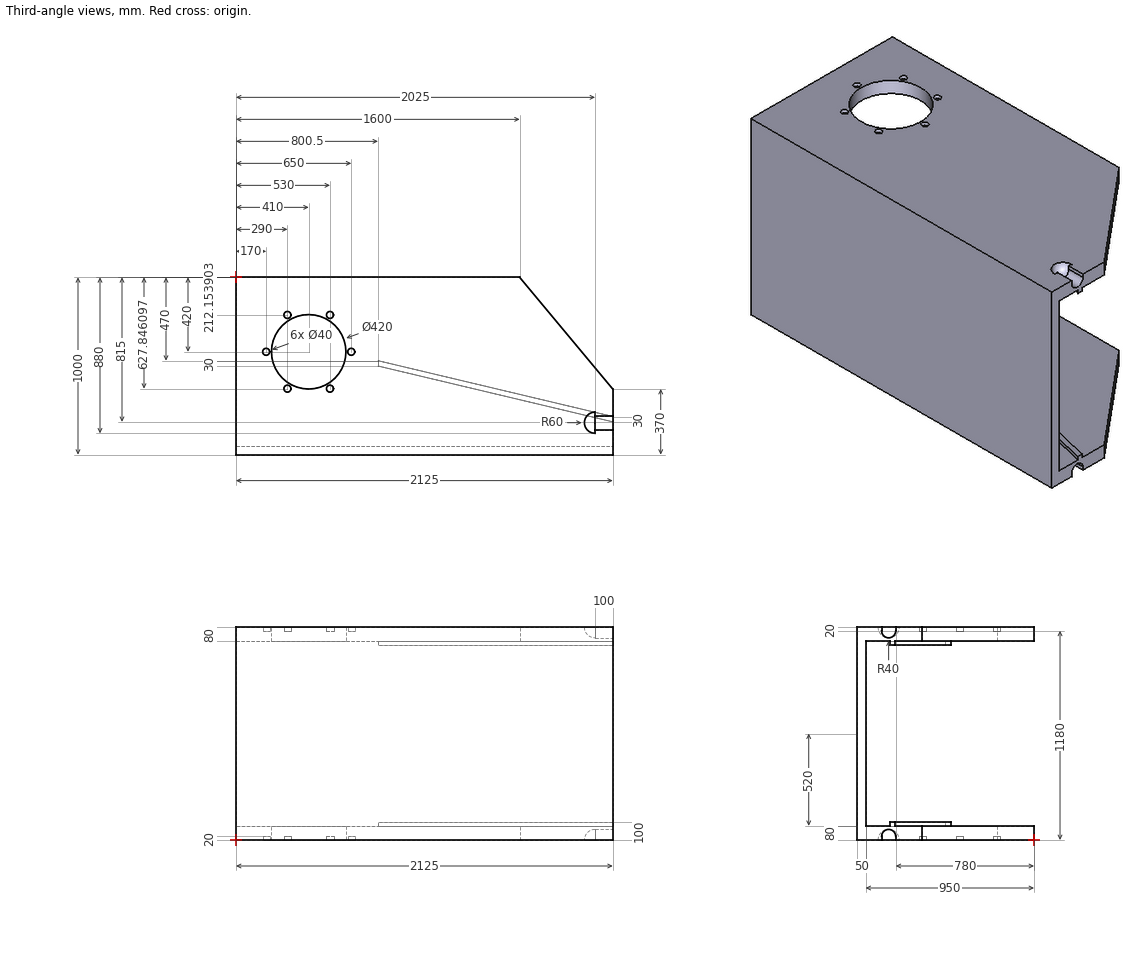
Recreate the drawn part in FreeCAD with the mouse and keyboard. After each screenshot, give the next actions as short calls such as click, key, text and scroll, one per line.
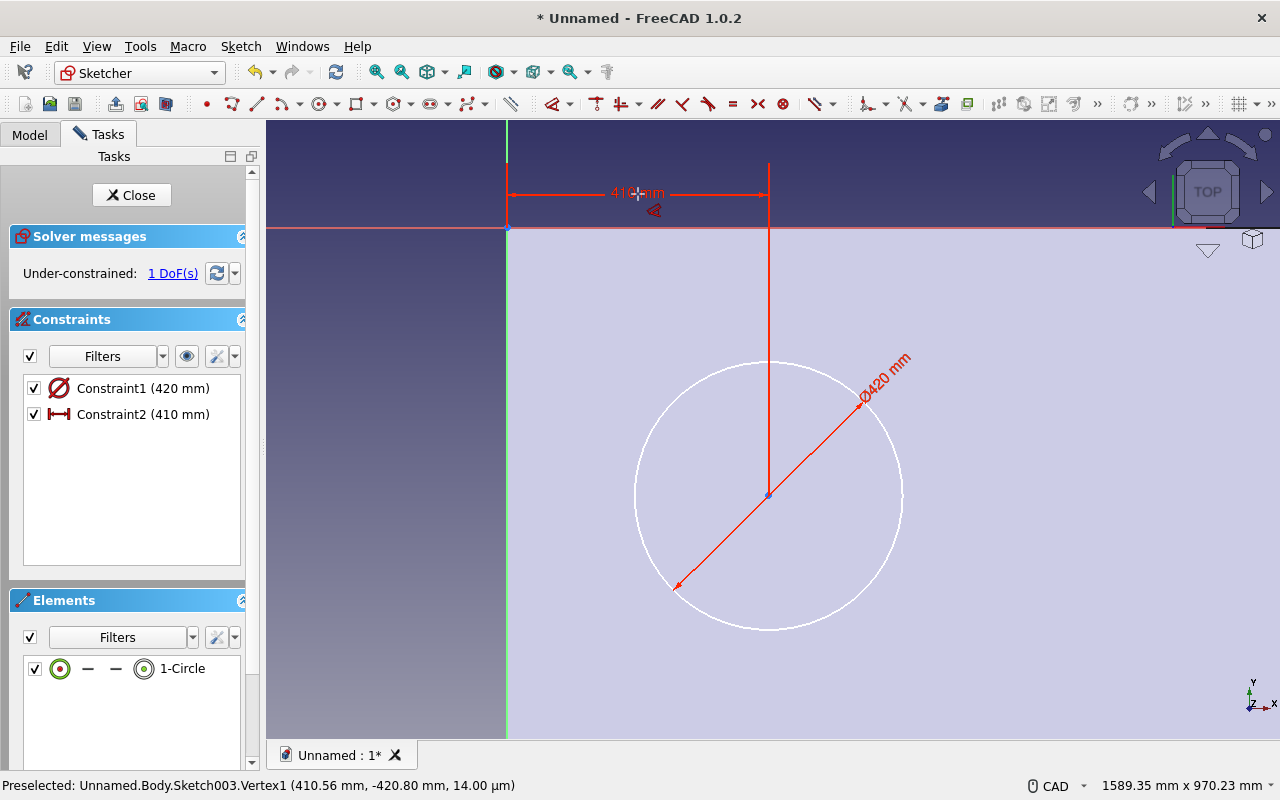
click(769, 496)
click(473, 362)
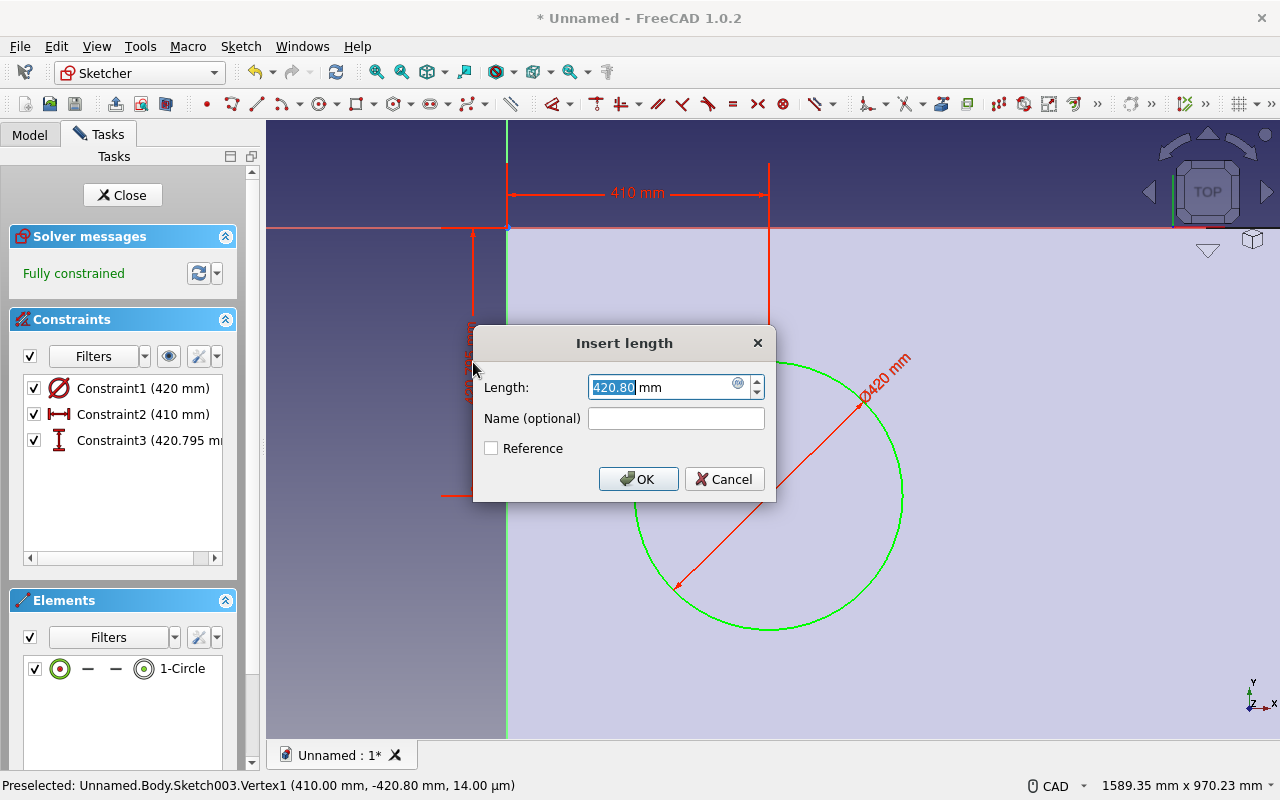
text(420)
key(Return)
key(Escape)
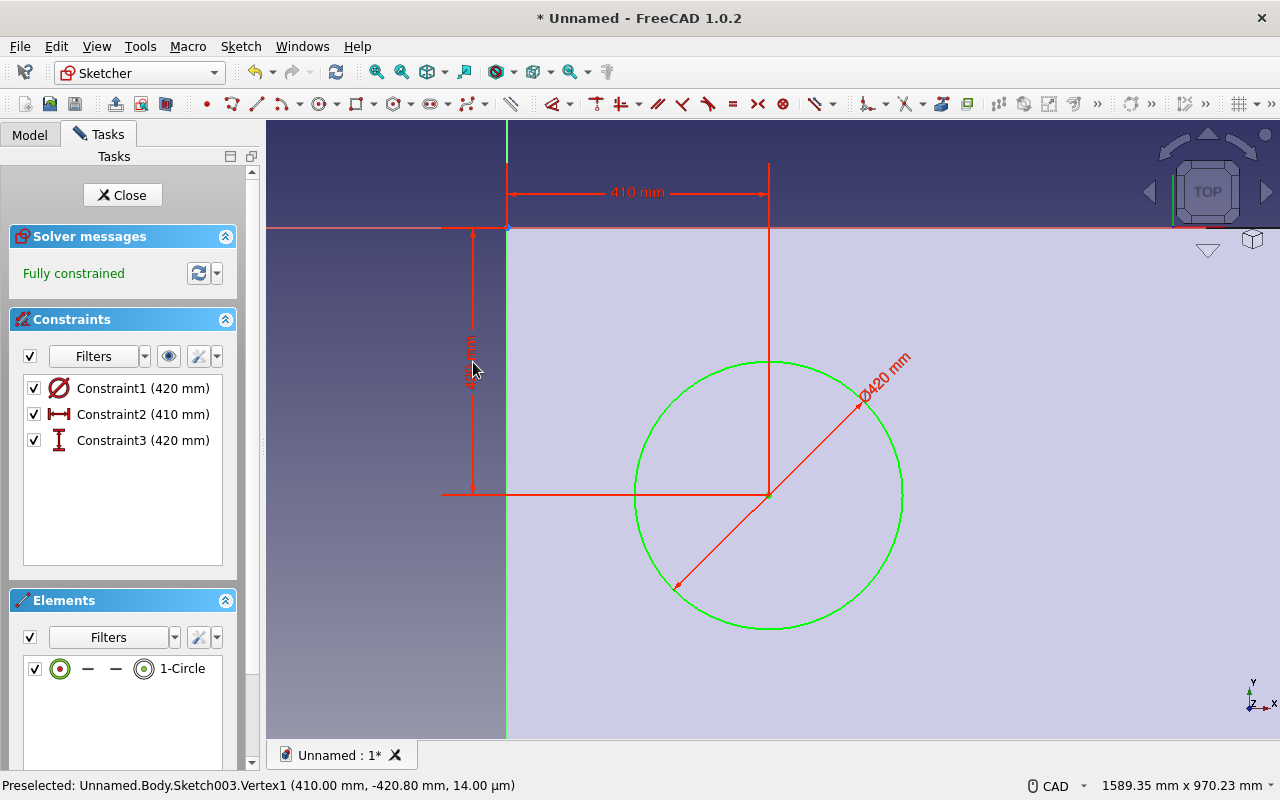
click(123, 195)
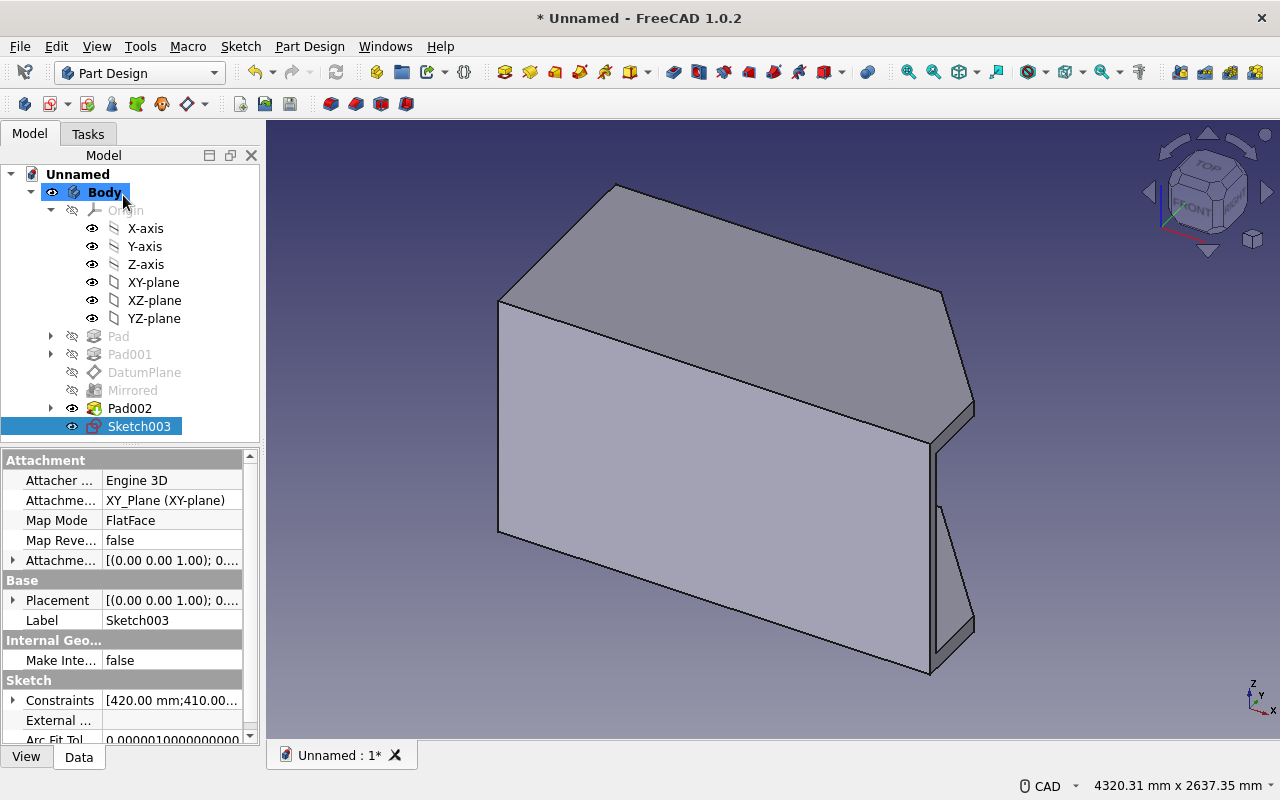
click(674, 72)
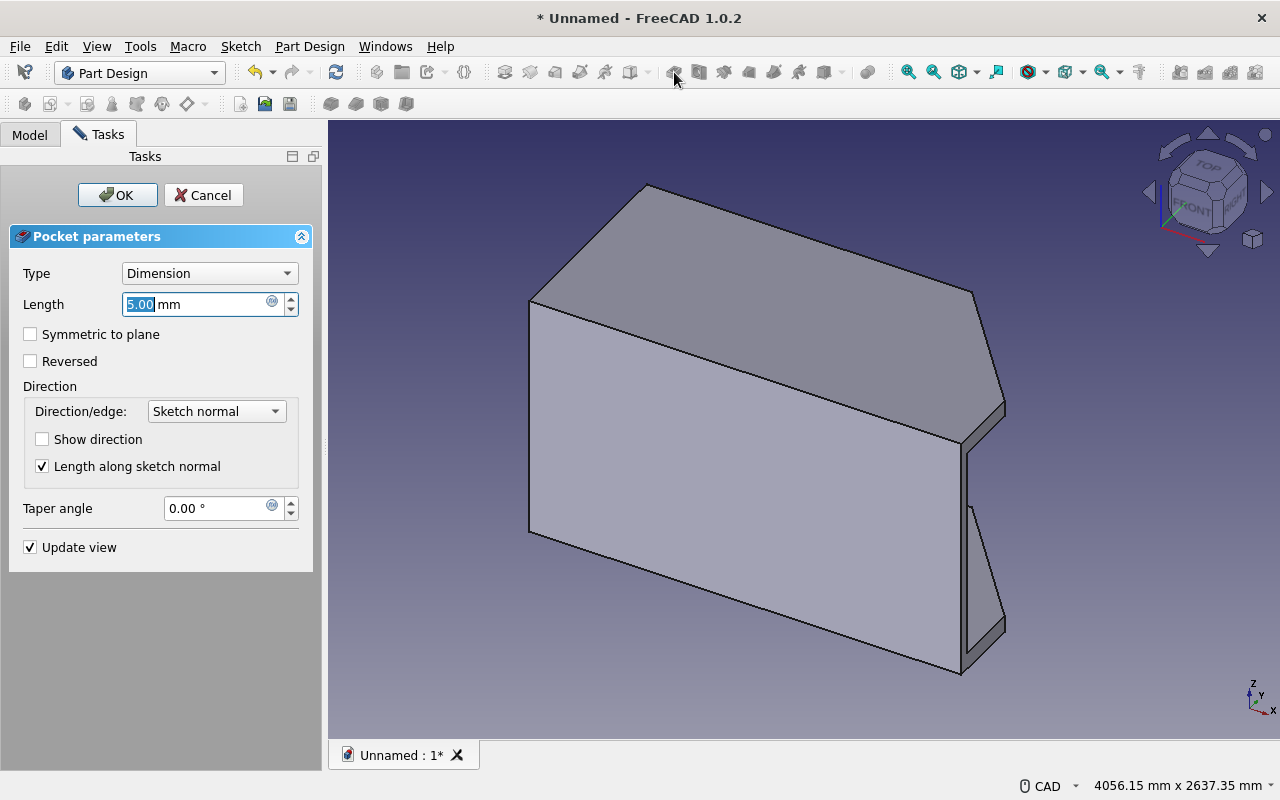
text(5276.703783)
key(Tab)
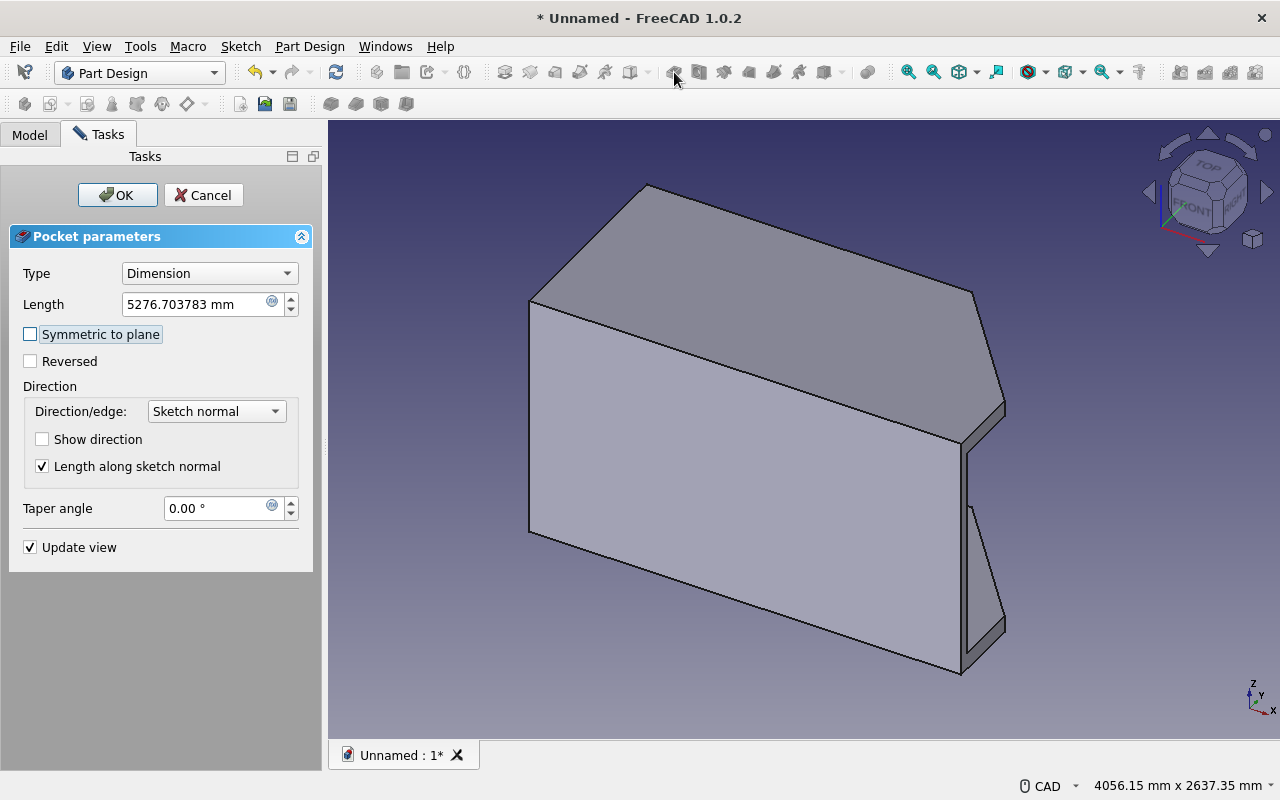
click(31, 334)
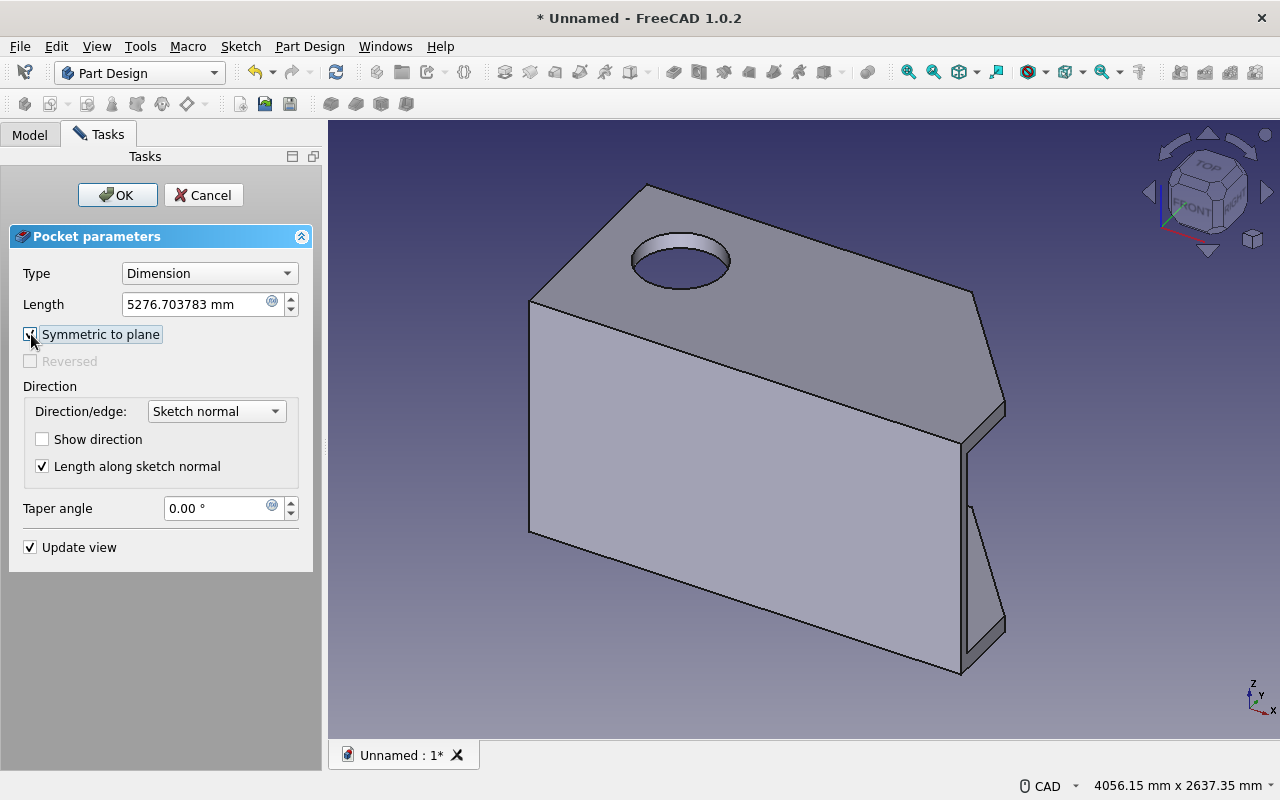
click(118, 195)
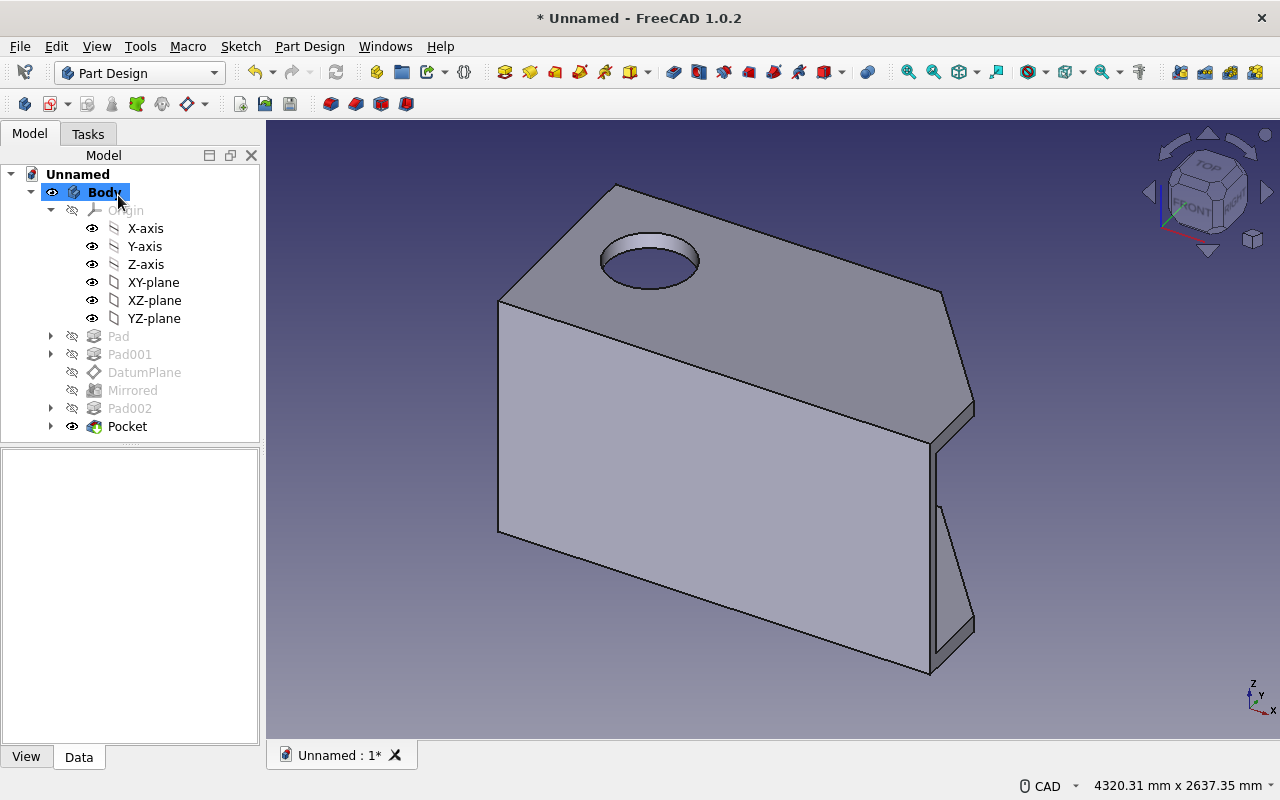
click(50, 104)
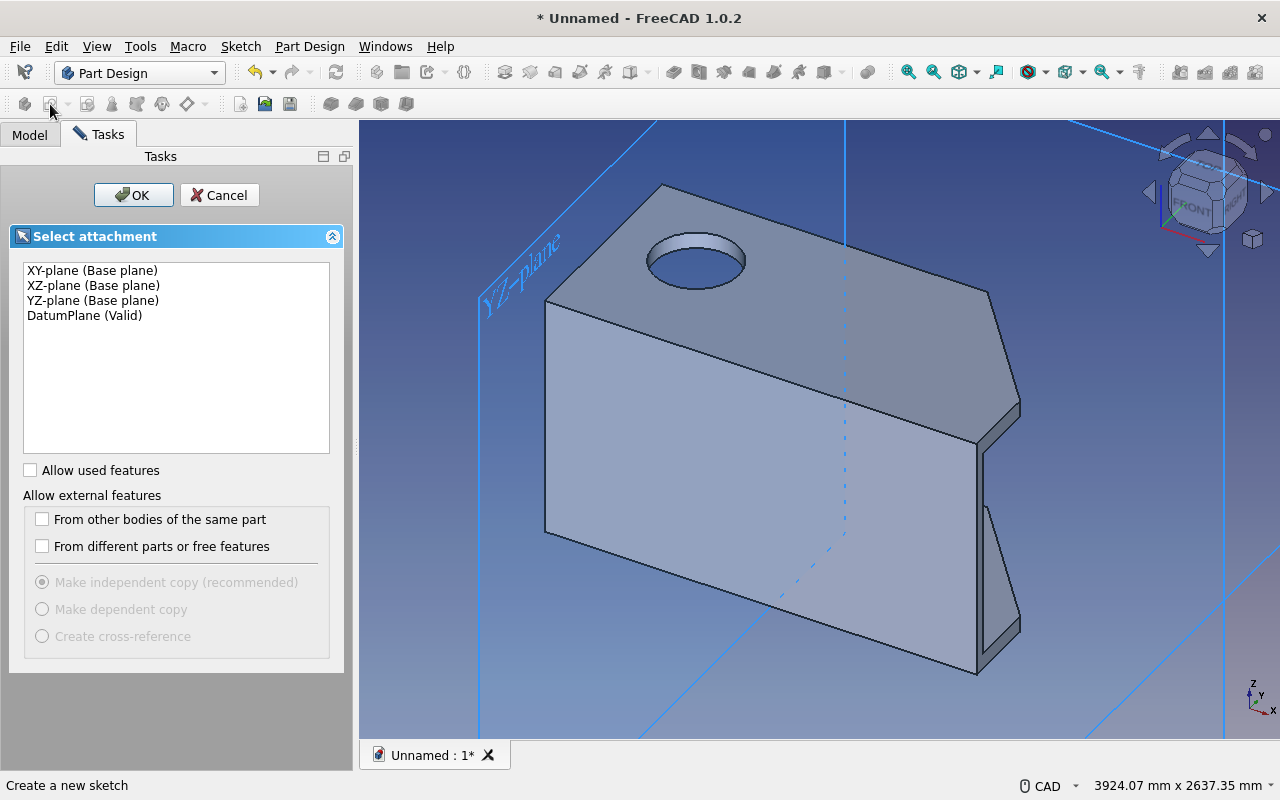
click(84, 270)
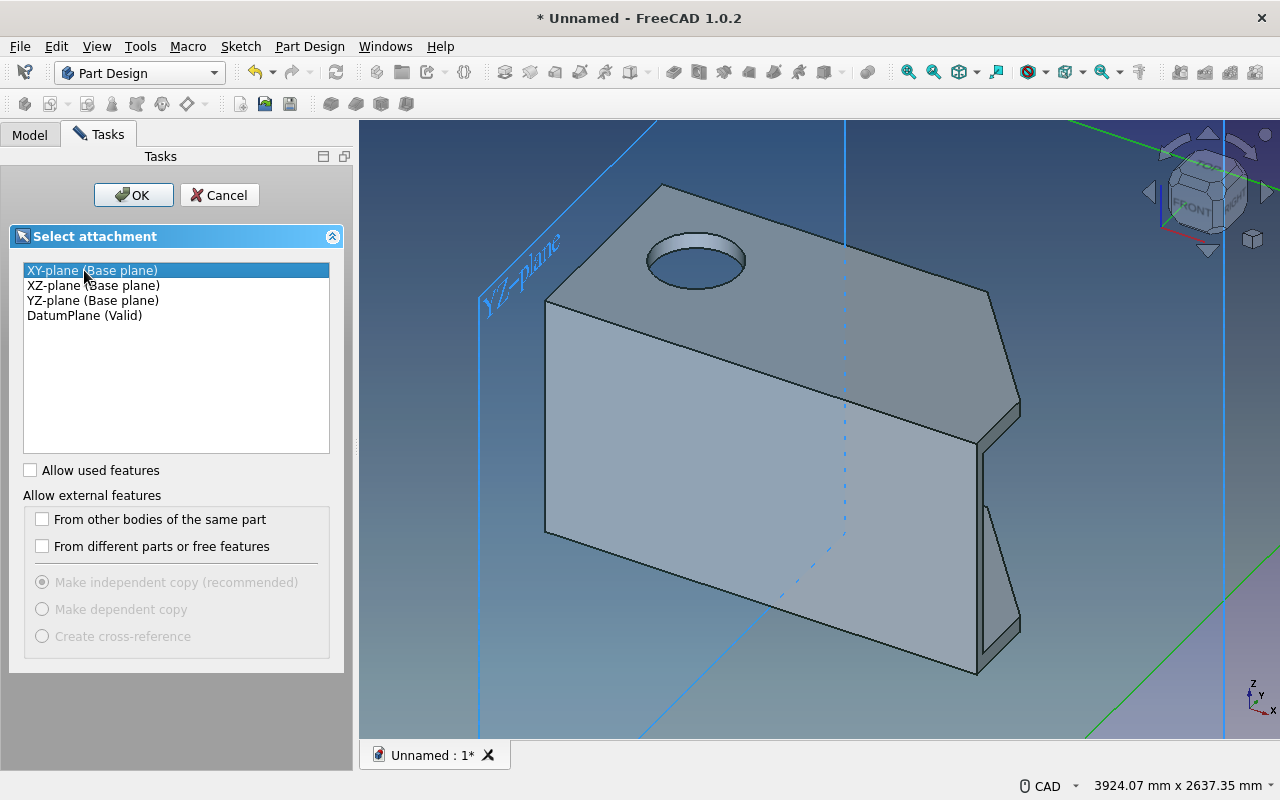
click(134, 195)